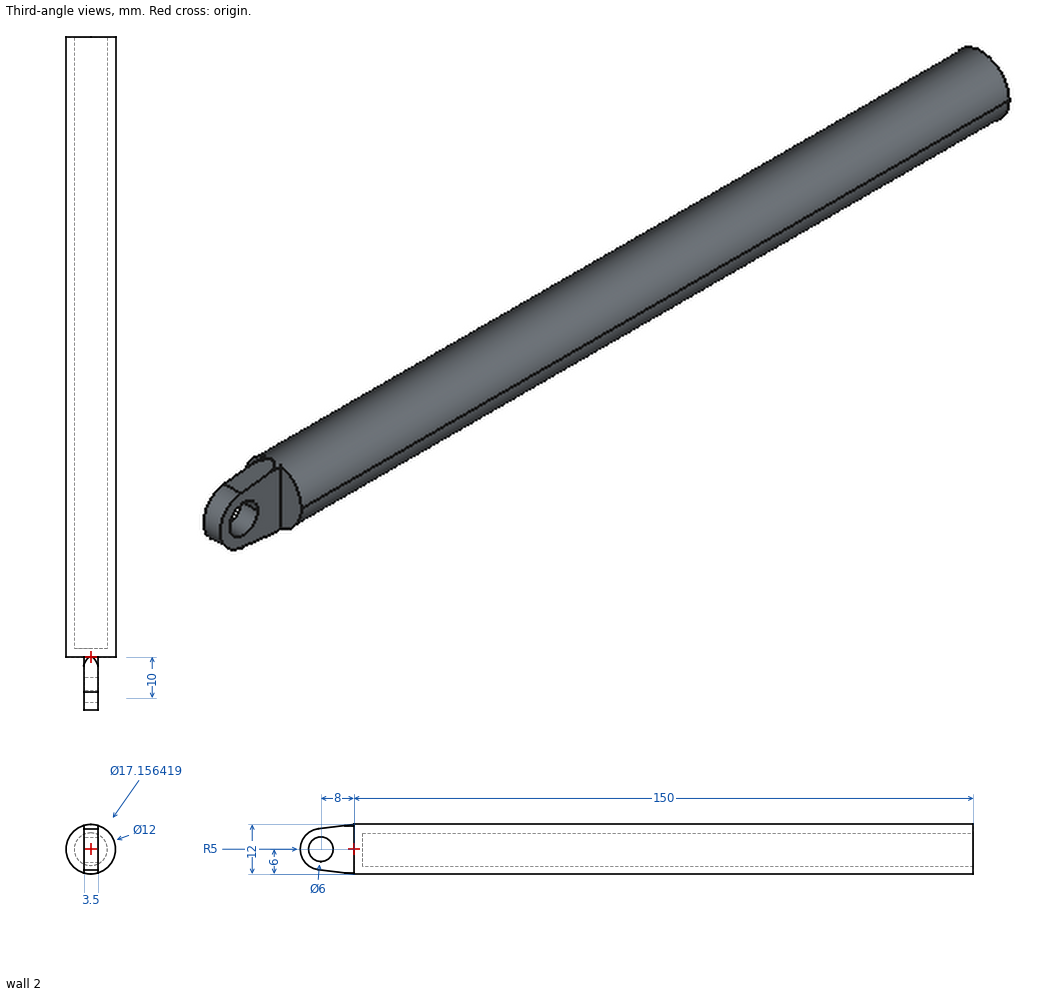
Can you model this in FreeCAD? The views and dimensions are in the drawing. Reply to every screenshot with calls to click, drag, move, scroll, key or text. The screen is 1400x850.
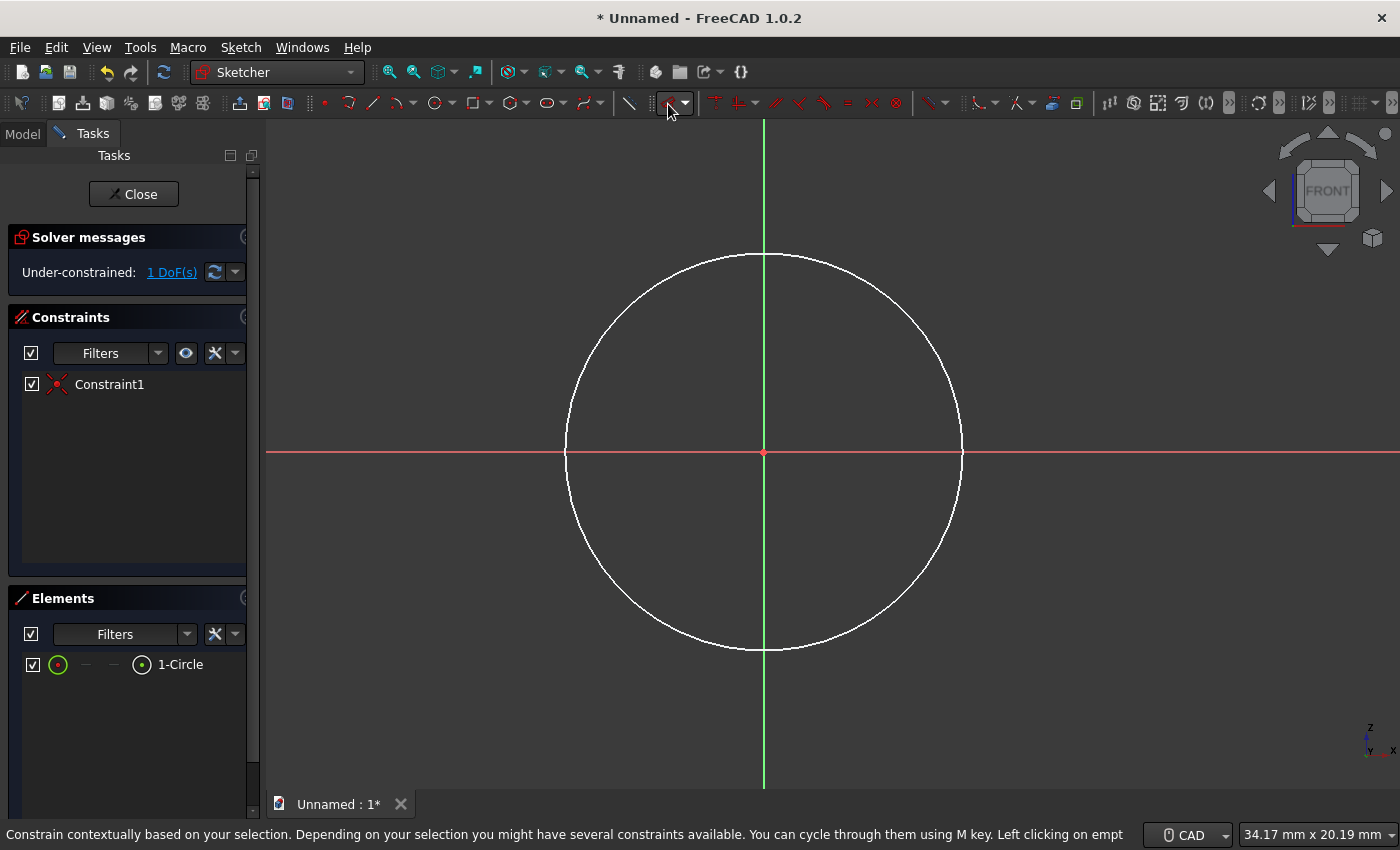
click(904, 311)
click(927, 288)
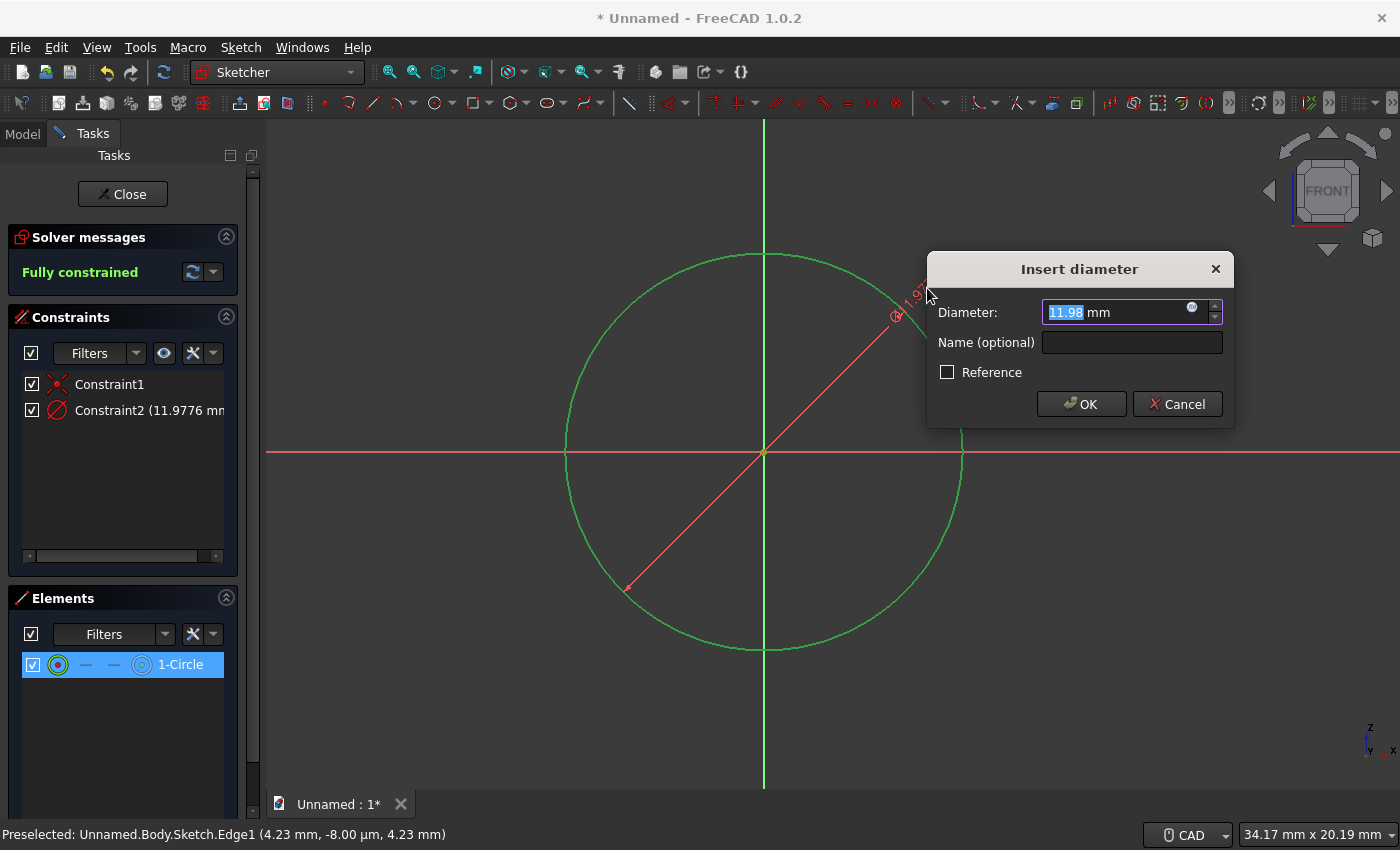
text(12)
key(Return)
key(Escape)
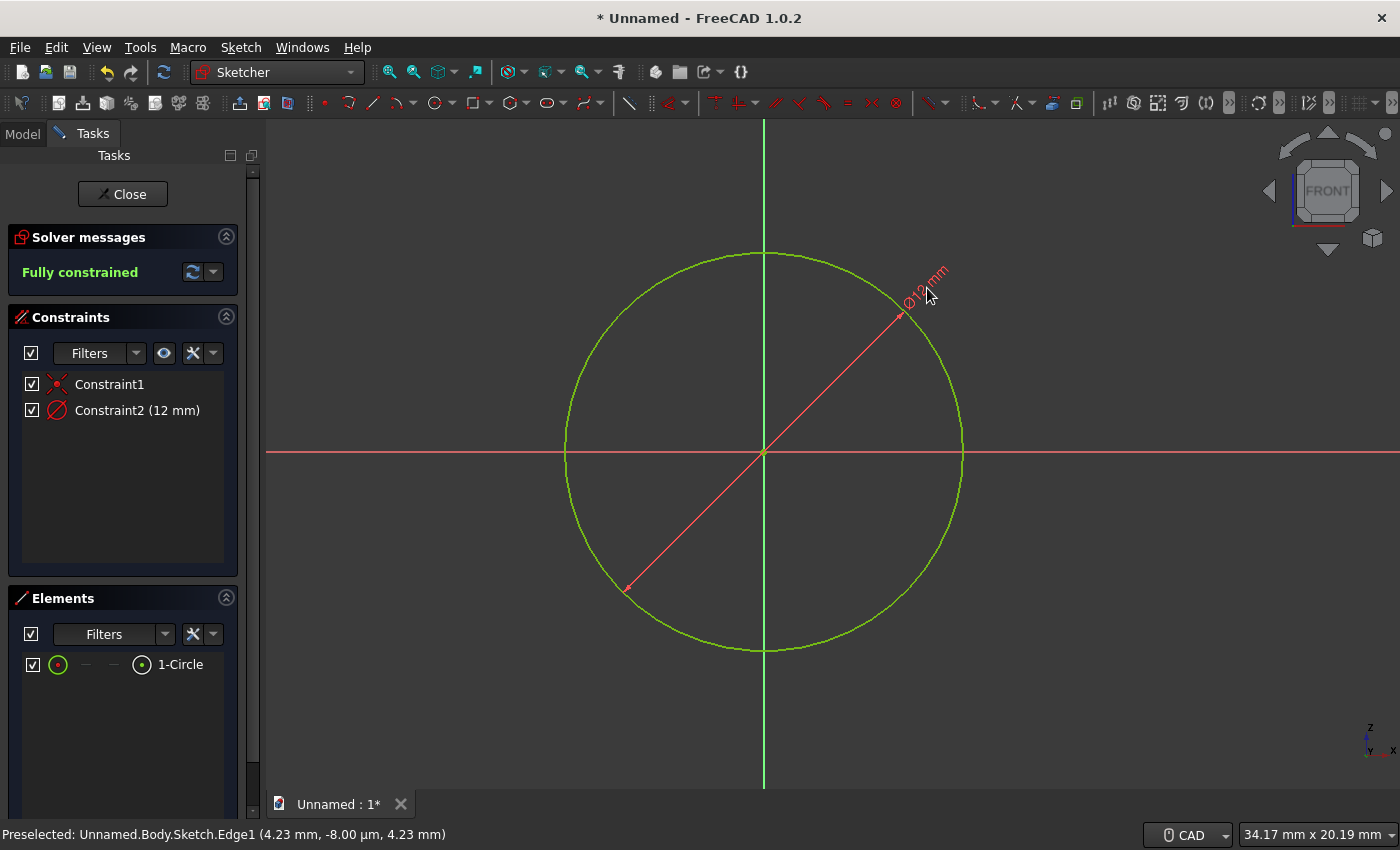
click(123, 194)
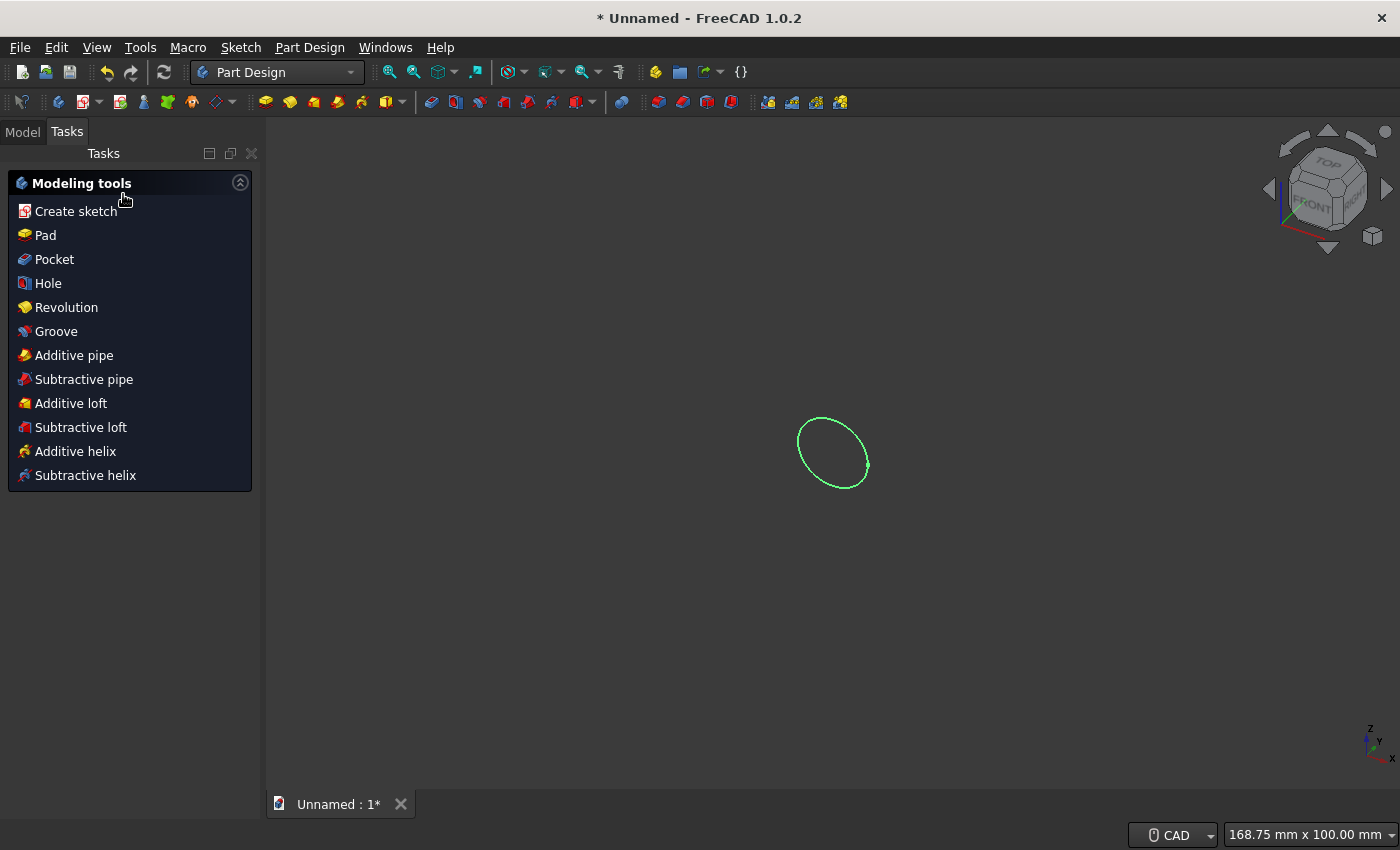
click(266, 102)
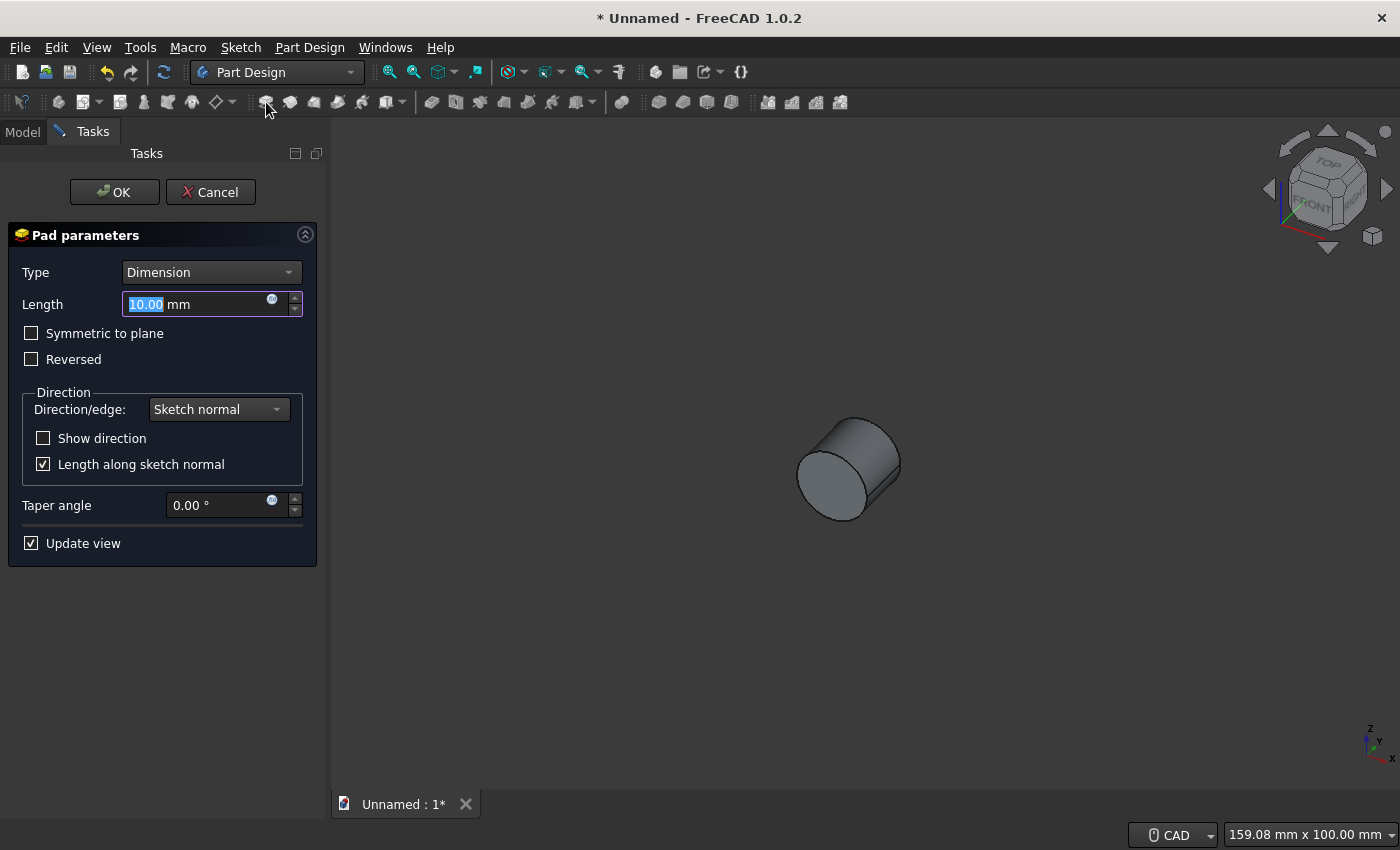
text(150)
key(Tab)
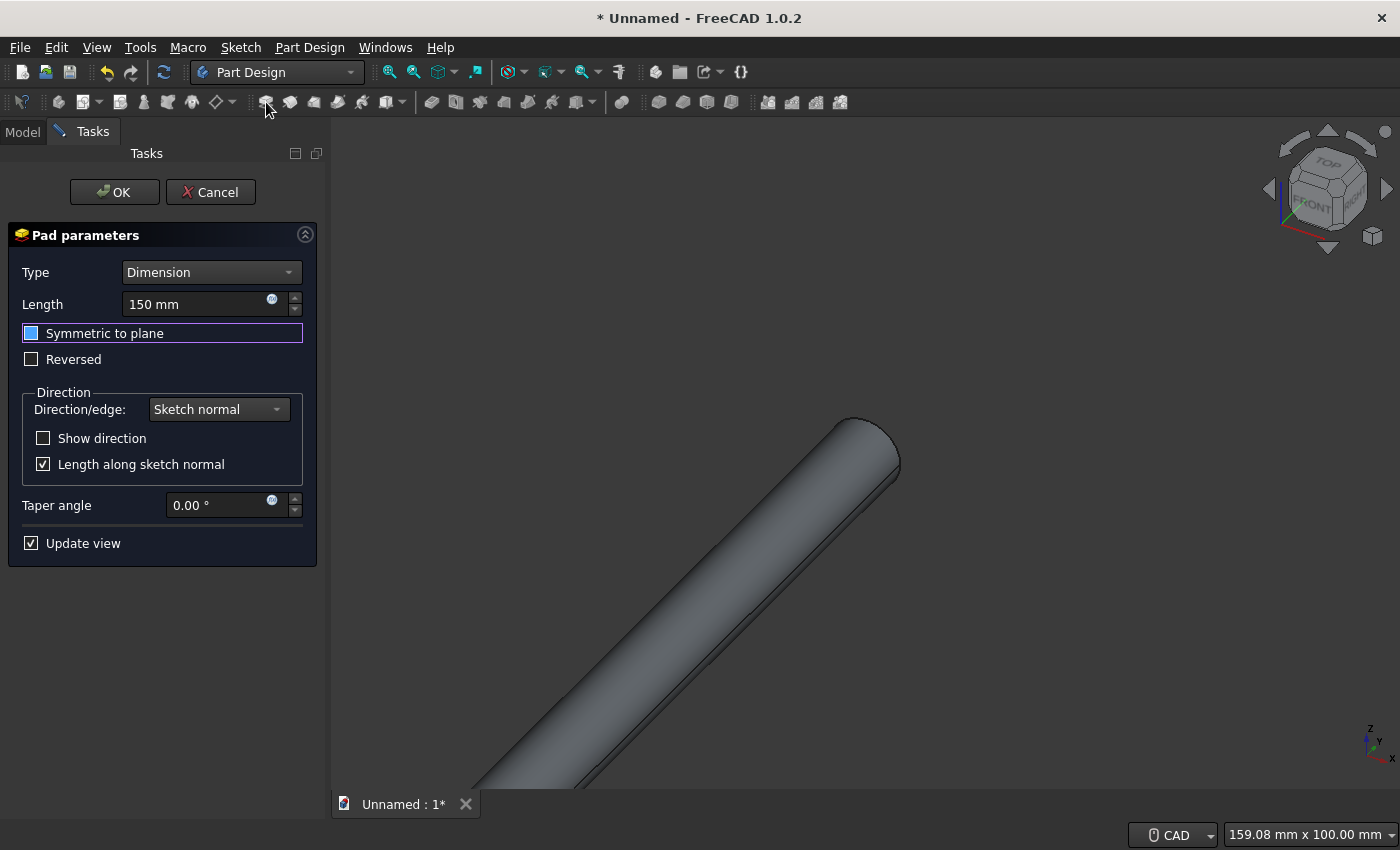
click(30, 359)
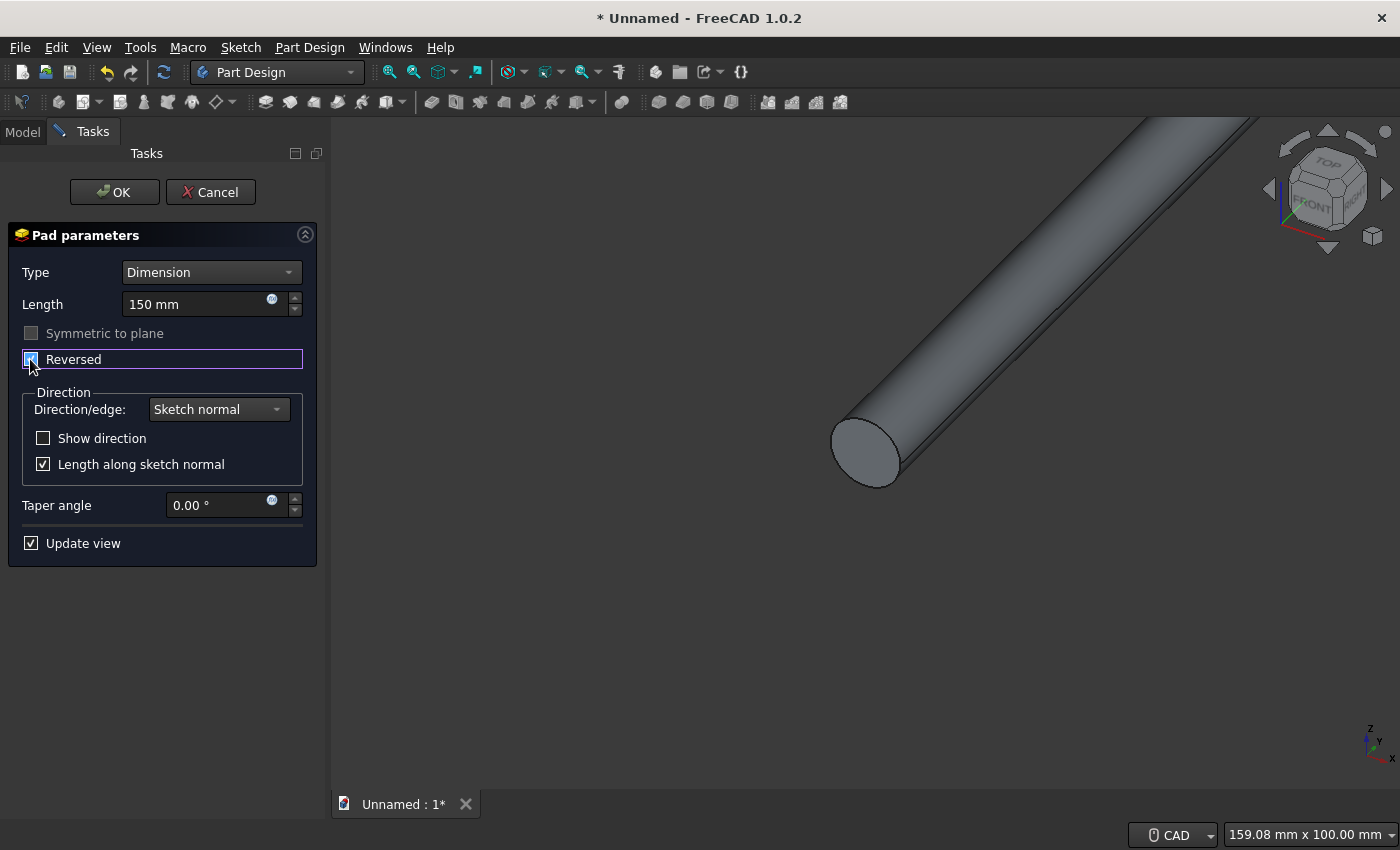
click(115, 192)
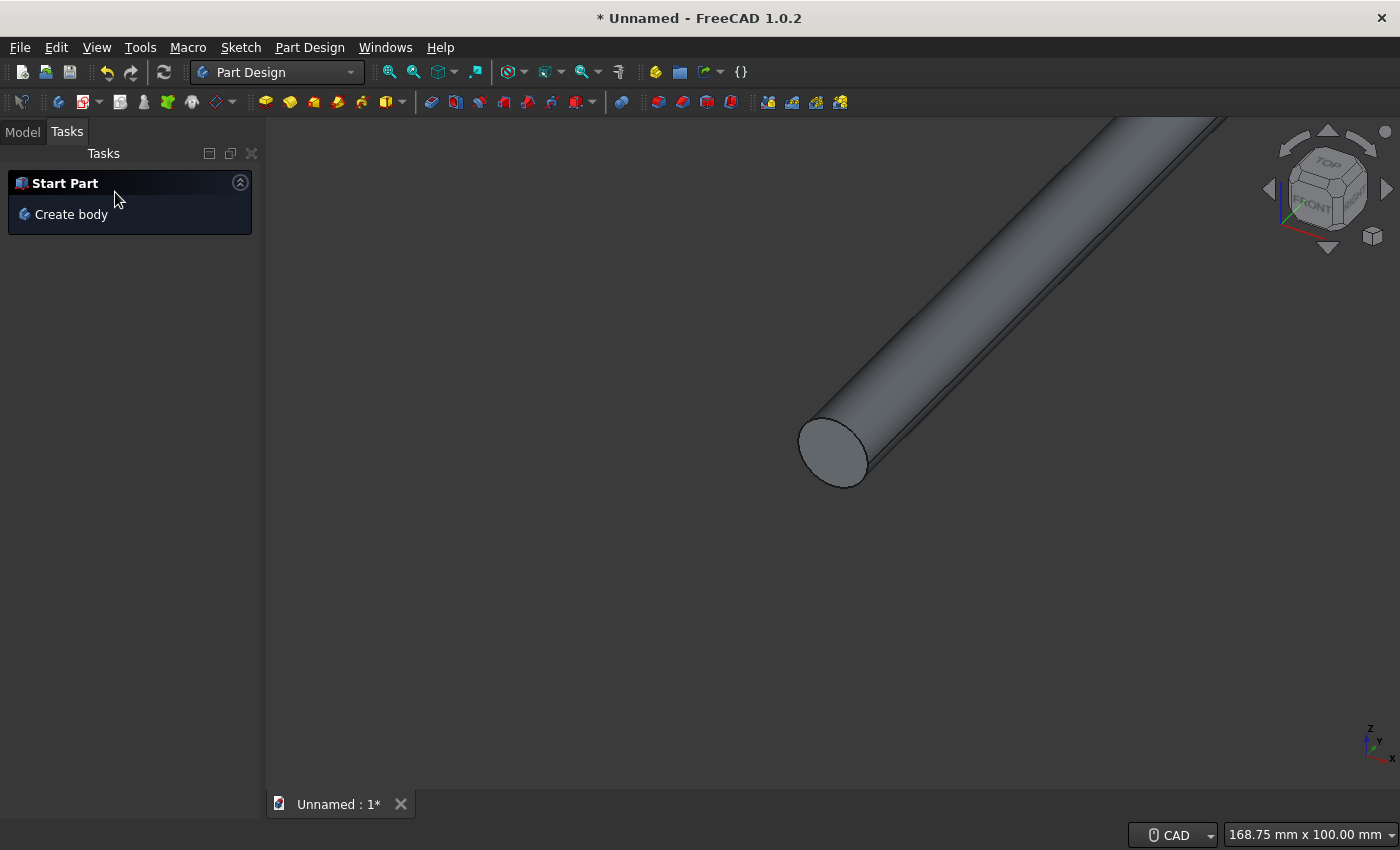
click(390, 72)